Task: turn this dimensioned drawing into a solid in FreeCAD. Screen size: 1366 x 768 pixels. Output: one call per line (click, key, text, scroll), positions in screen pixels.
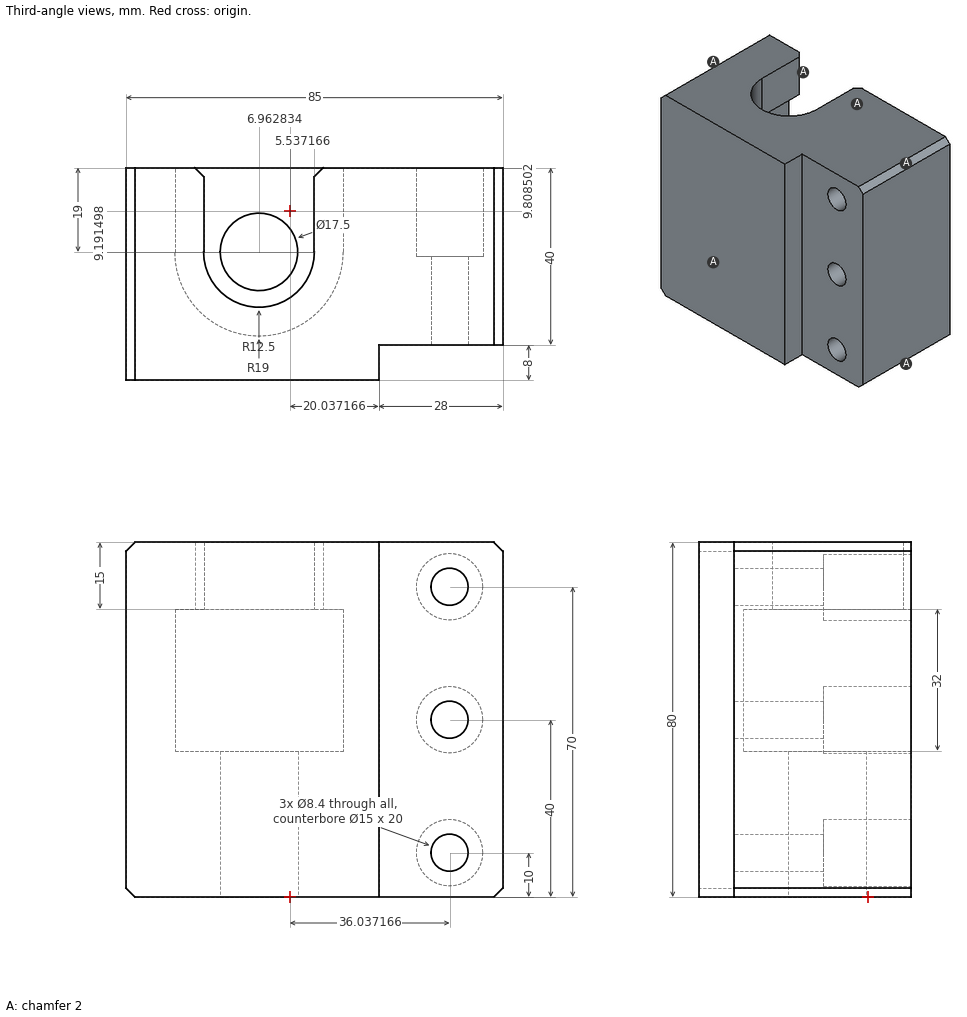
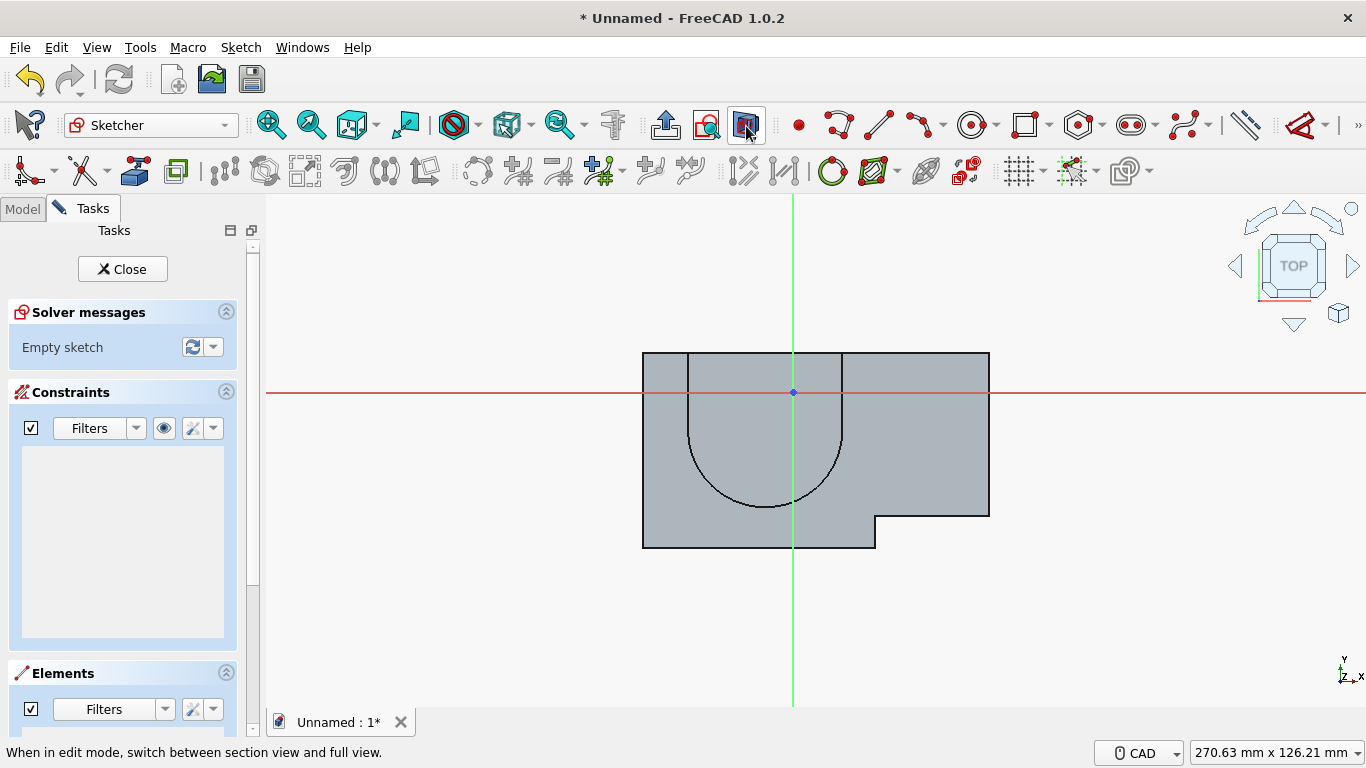
scroll(771, 422, up, 7)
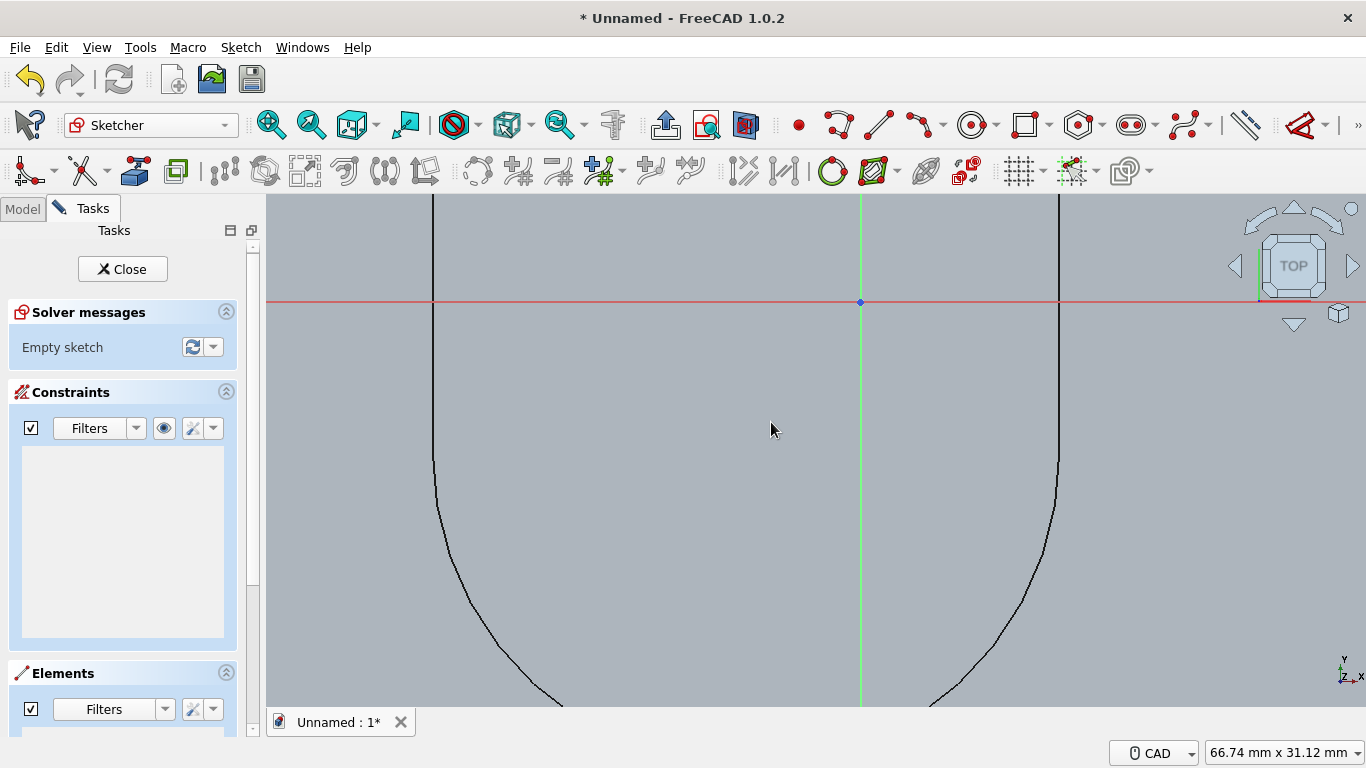
key(g)
key(c)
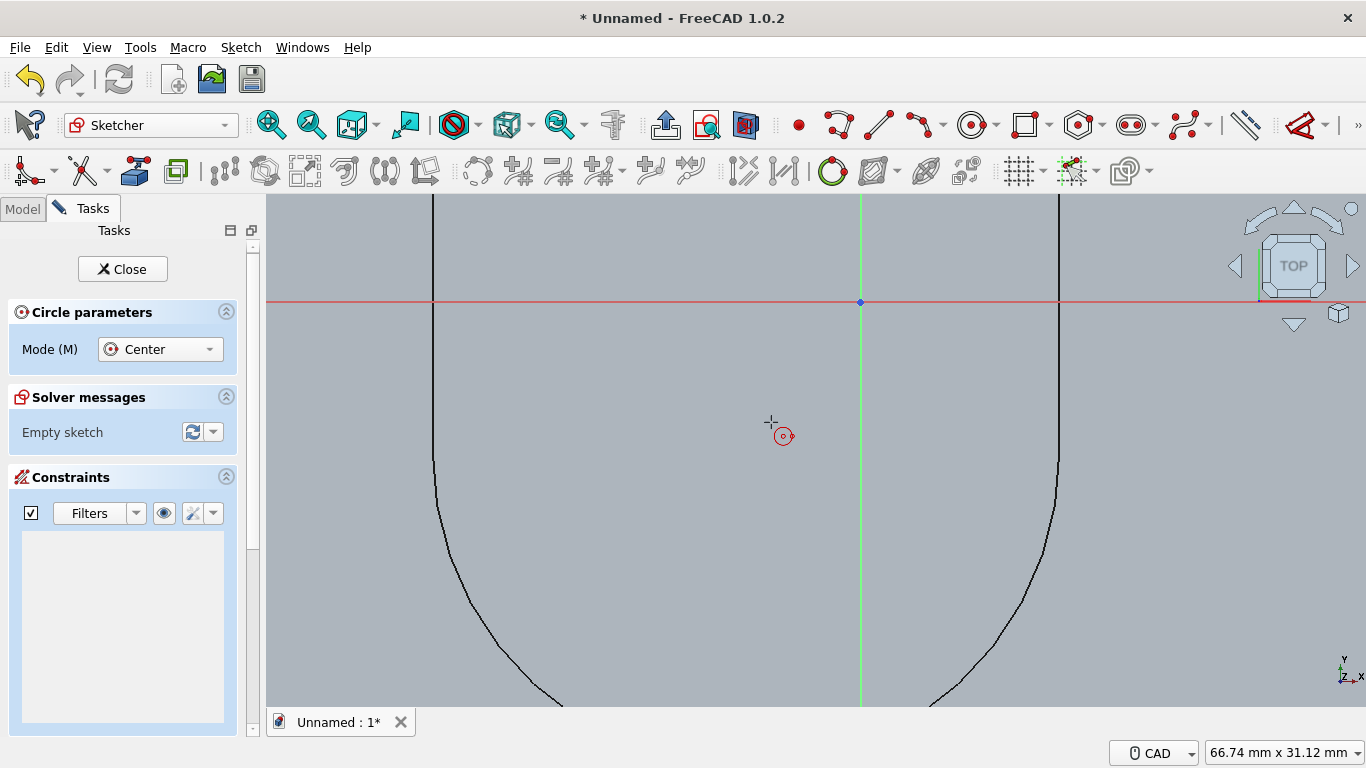
click(746, 454)
move(644, 352)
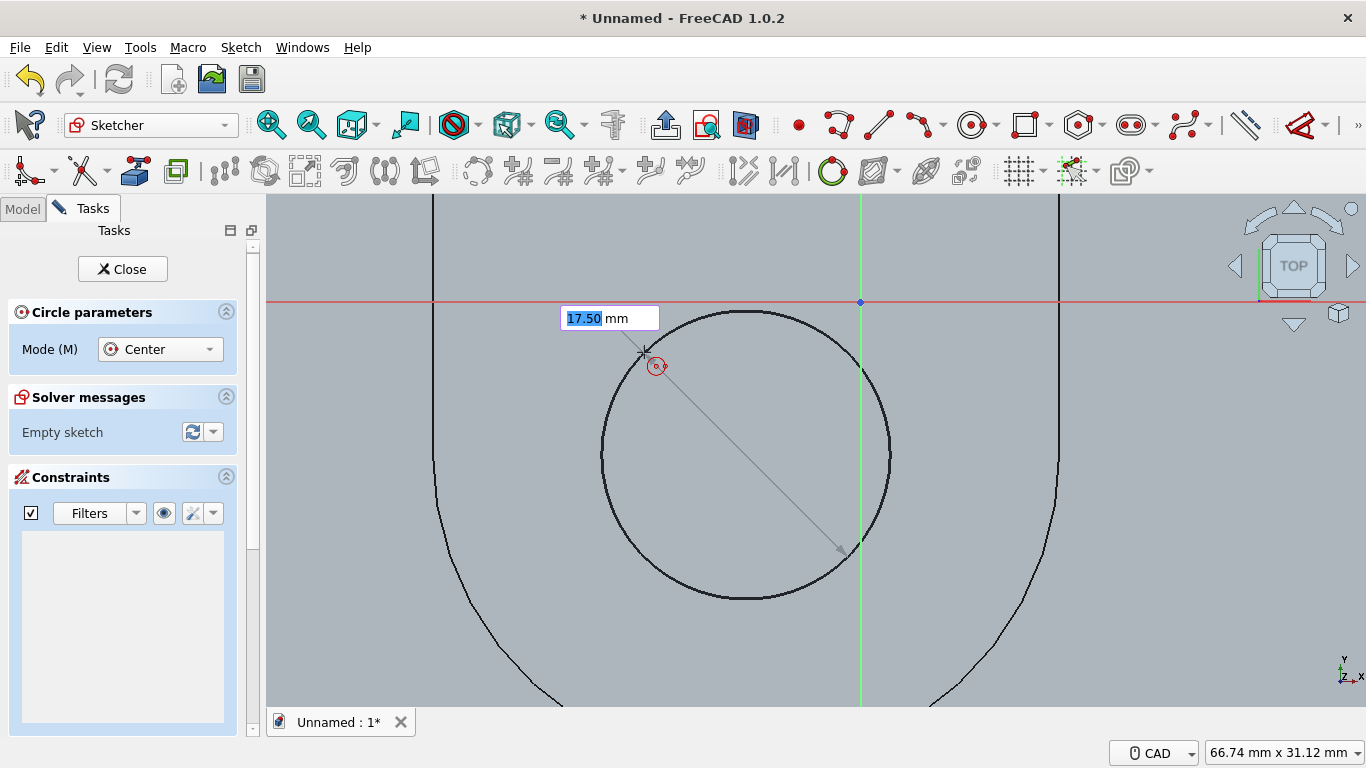
text(17.5)
key(Return)
key(Escape)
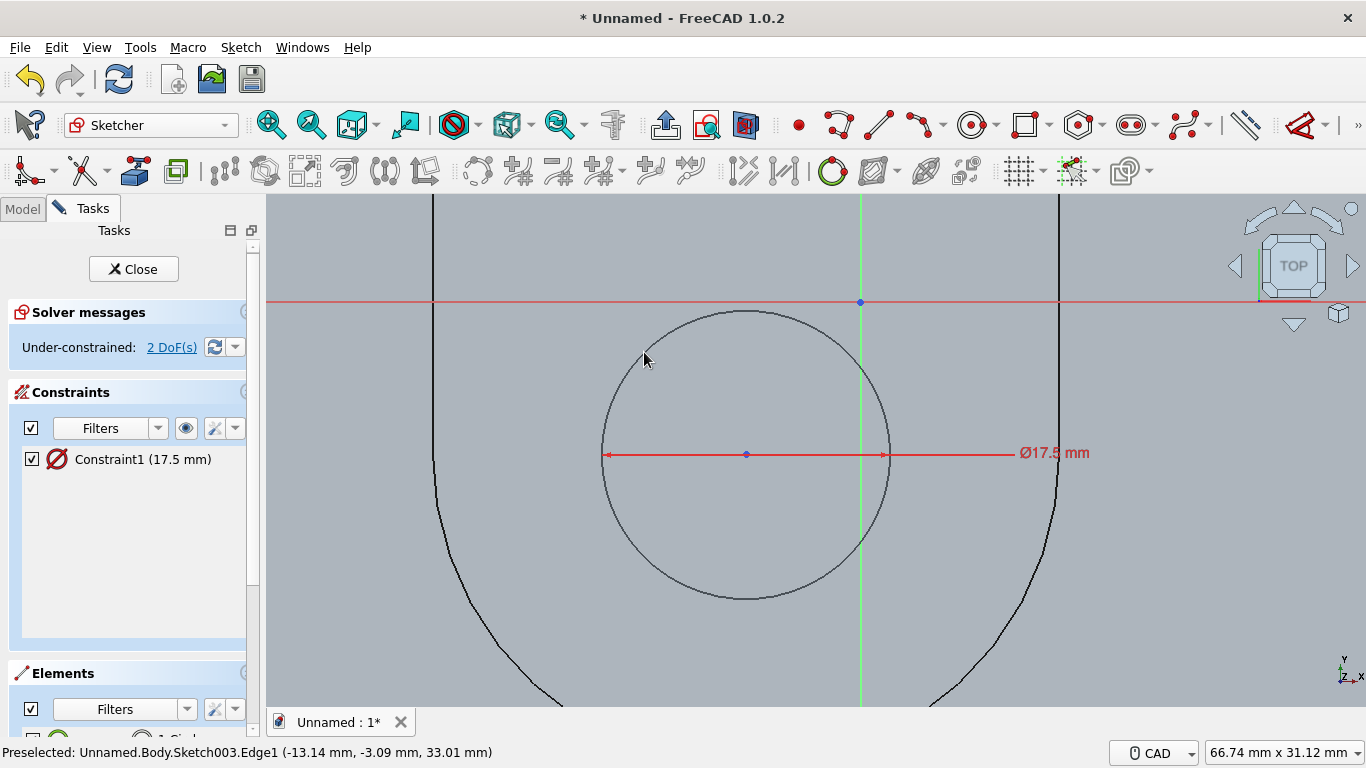
click(1300, 126)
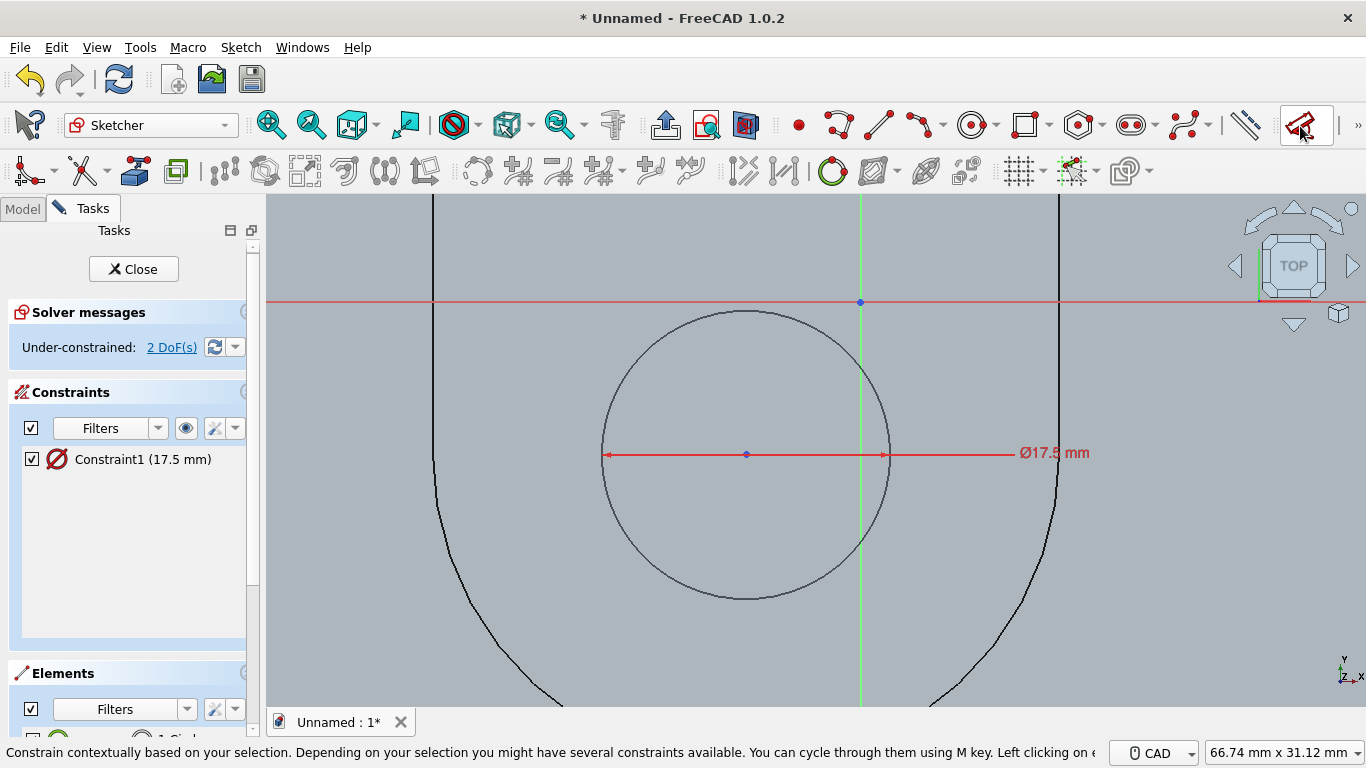
click(746, 455)
click(803, 268)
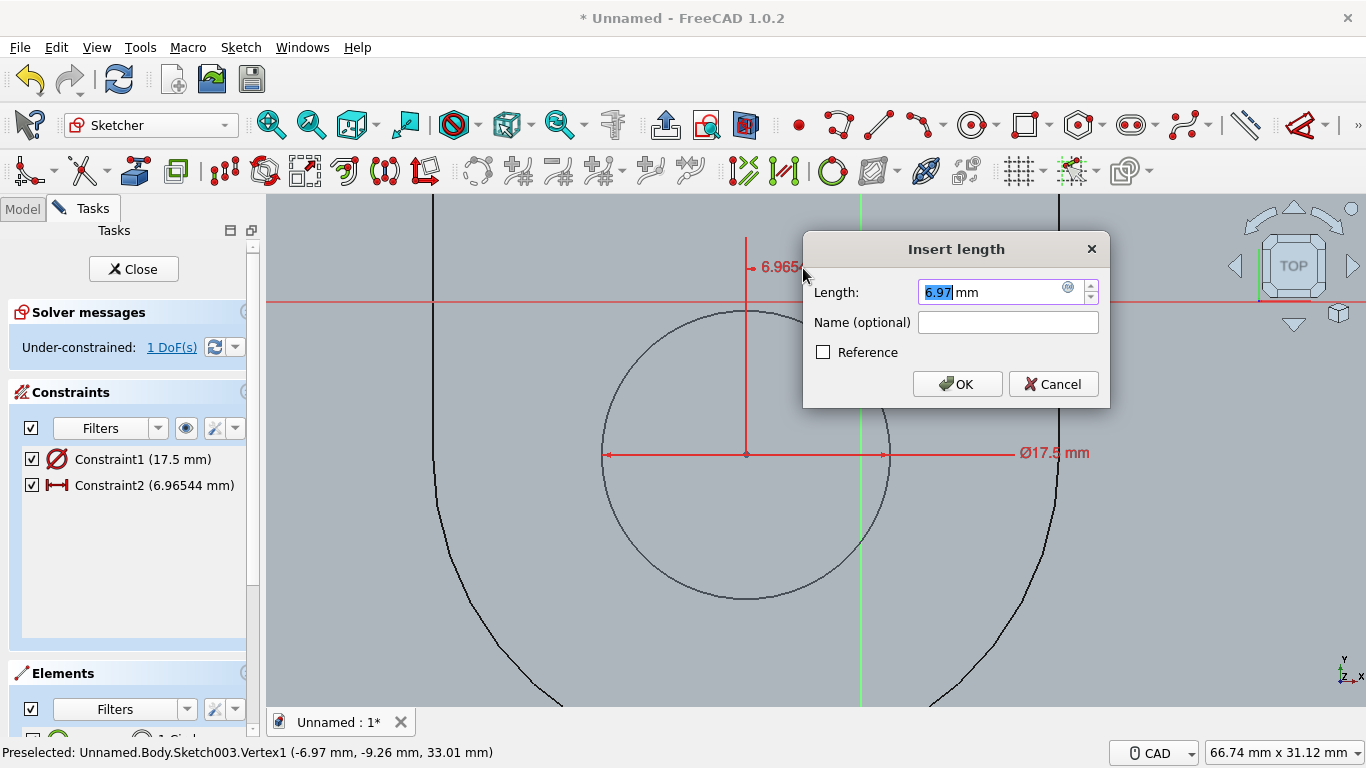
text(6.962834)
key(Return)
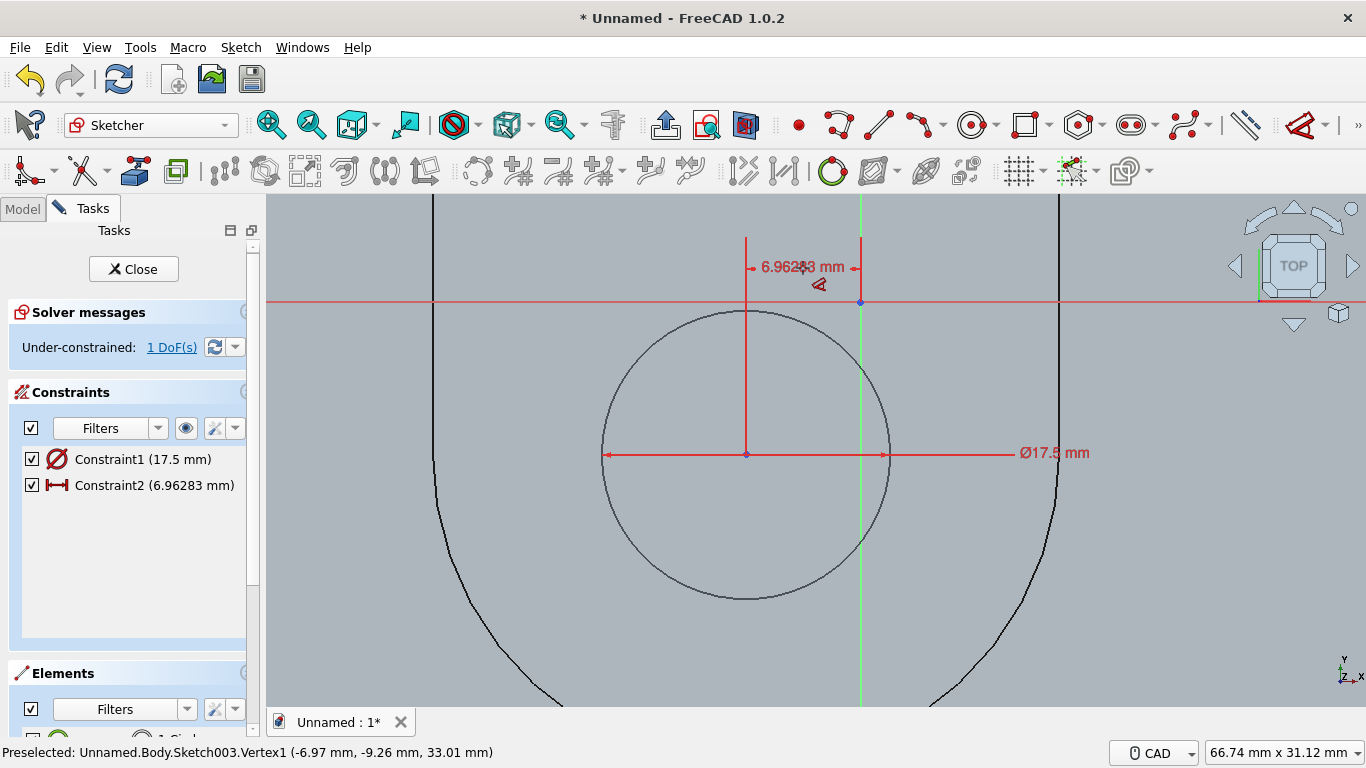
click(746, 455)
click(895, 379)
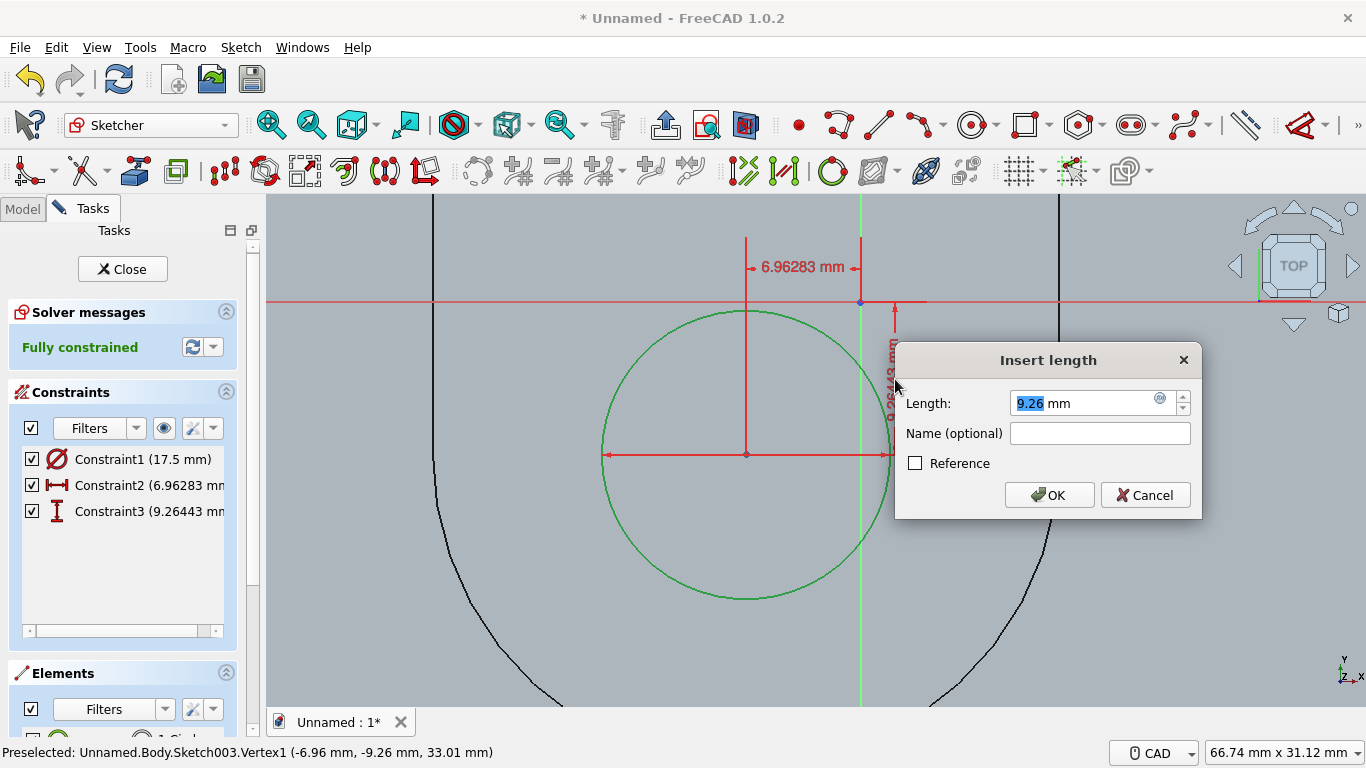
text(9.191498)
key(Return)
key(Escape)